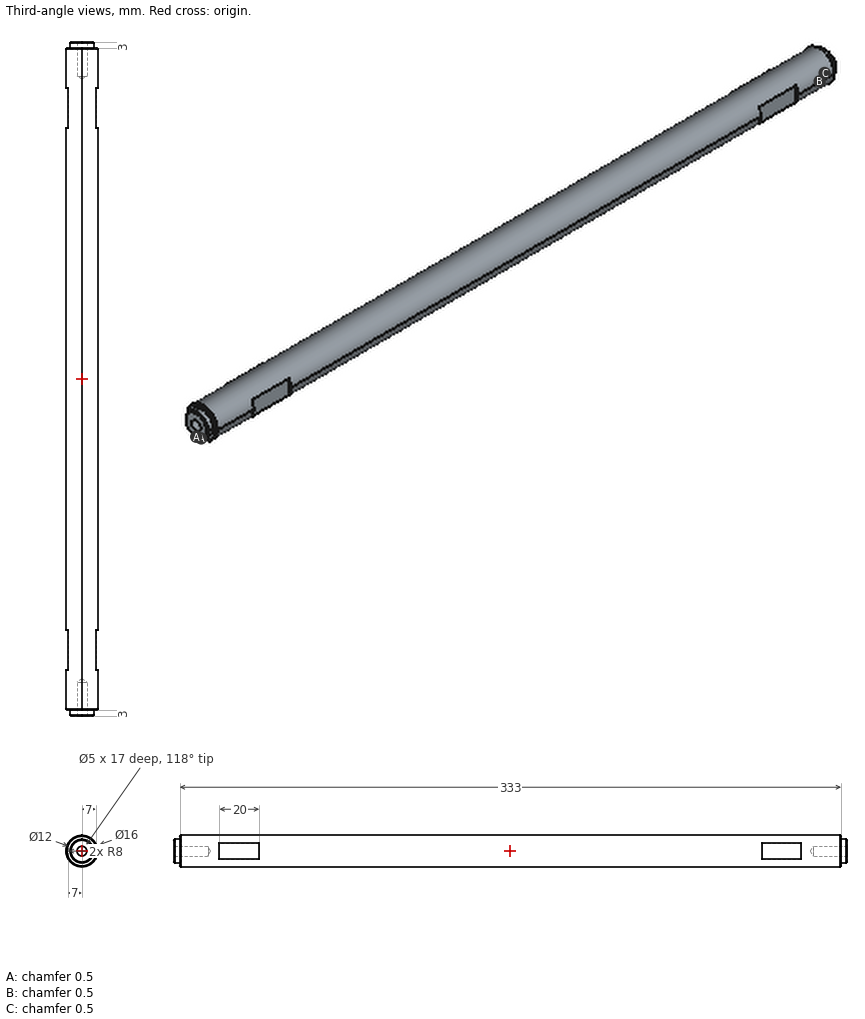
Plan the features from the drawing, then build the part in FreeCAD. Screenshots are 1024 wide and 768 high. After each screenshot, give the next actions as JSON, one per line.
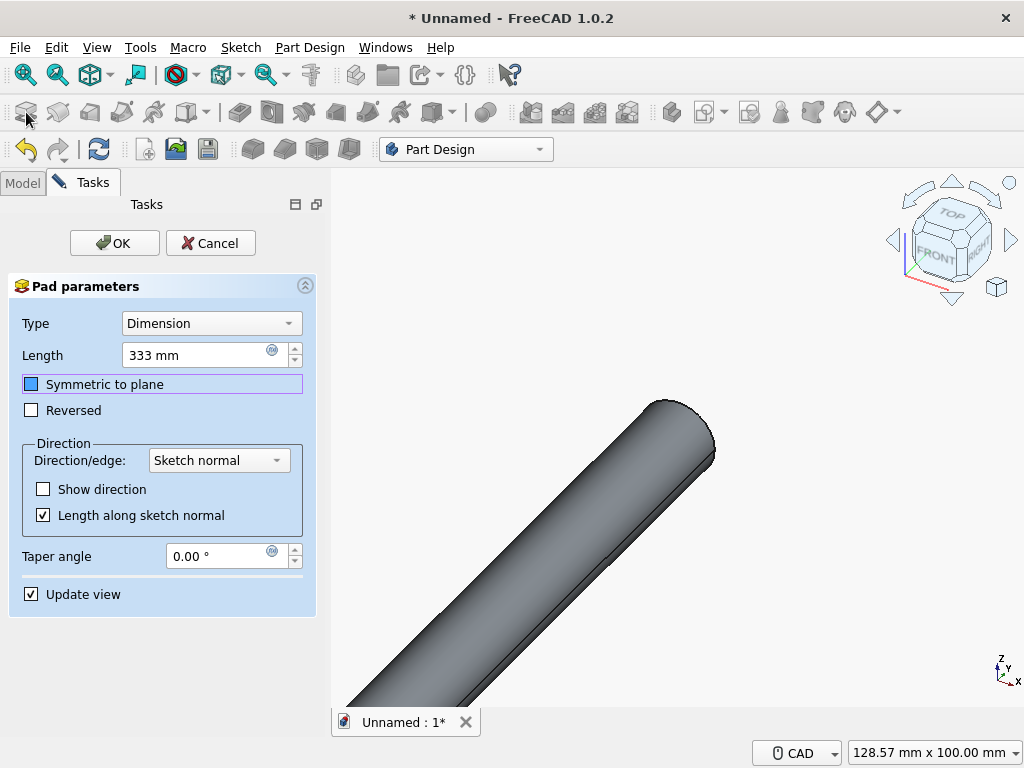
{"action": "left_click", "coordinate": [30, 384]}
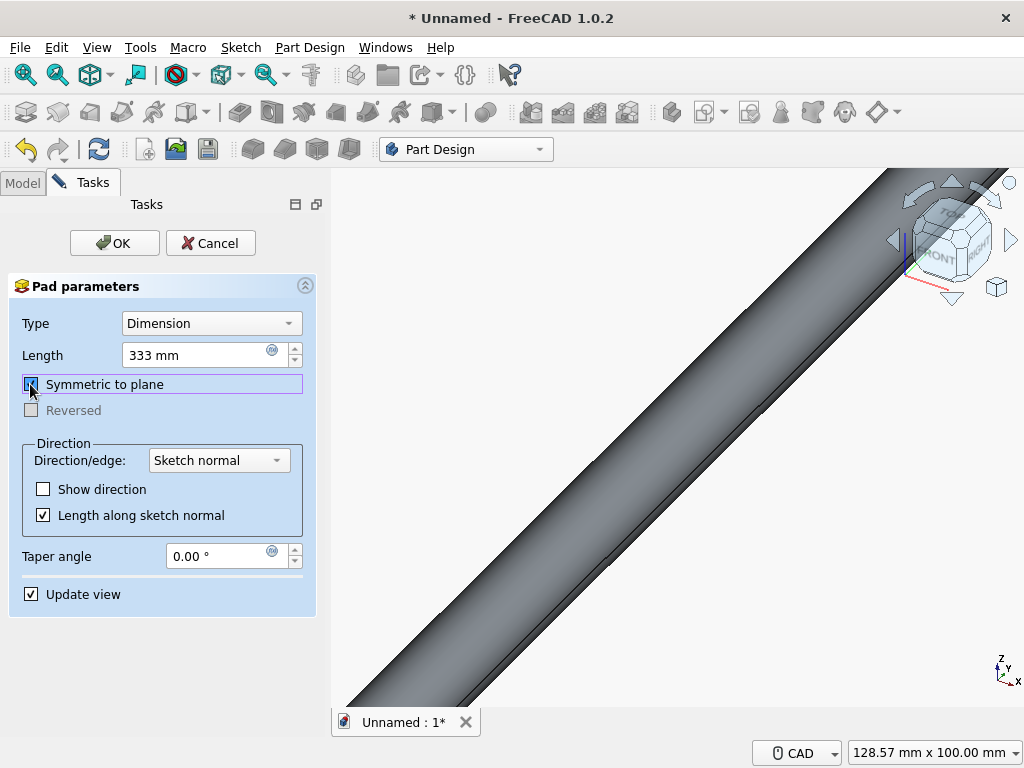
{"action": "left_click", "coordinate": [115, 243]}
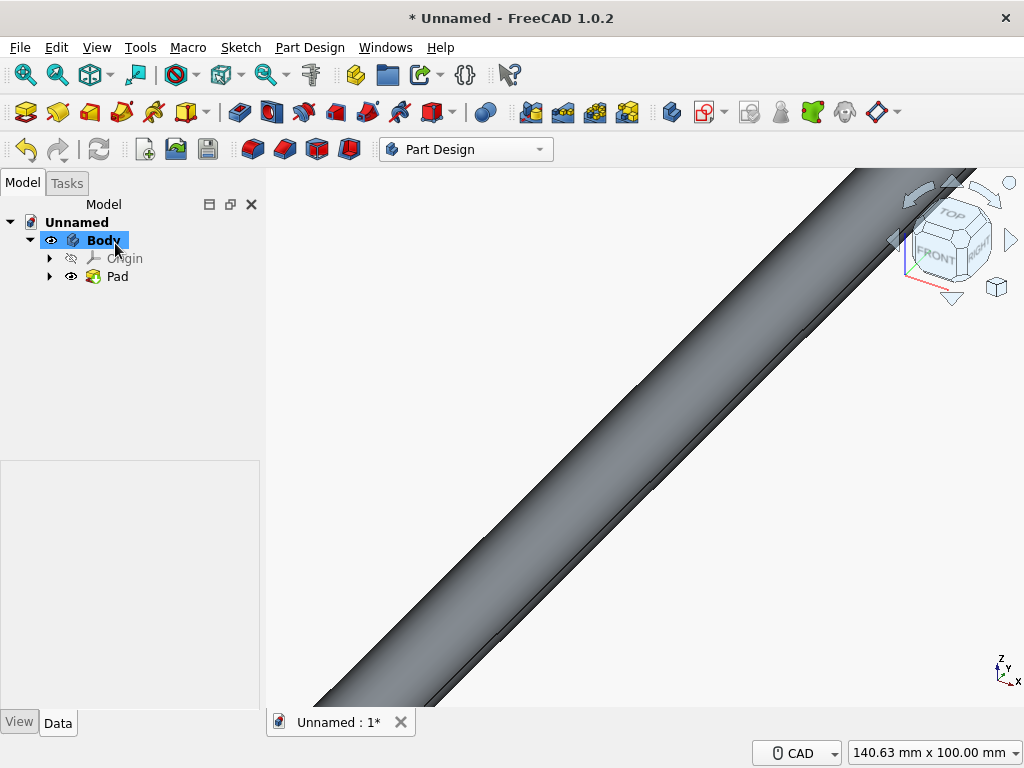
{"action": "left_click", "coordinate": [26, 76]}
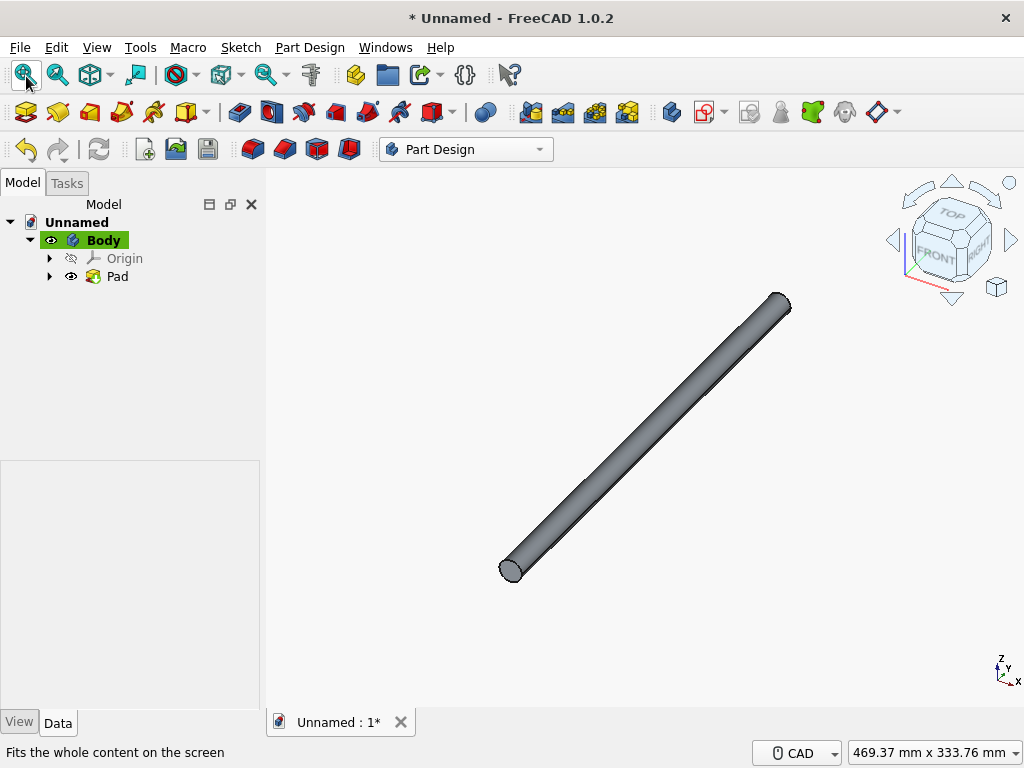
{"action": "left_click", "coordinate": [511, 573]}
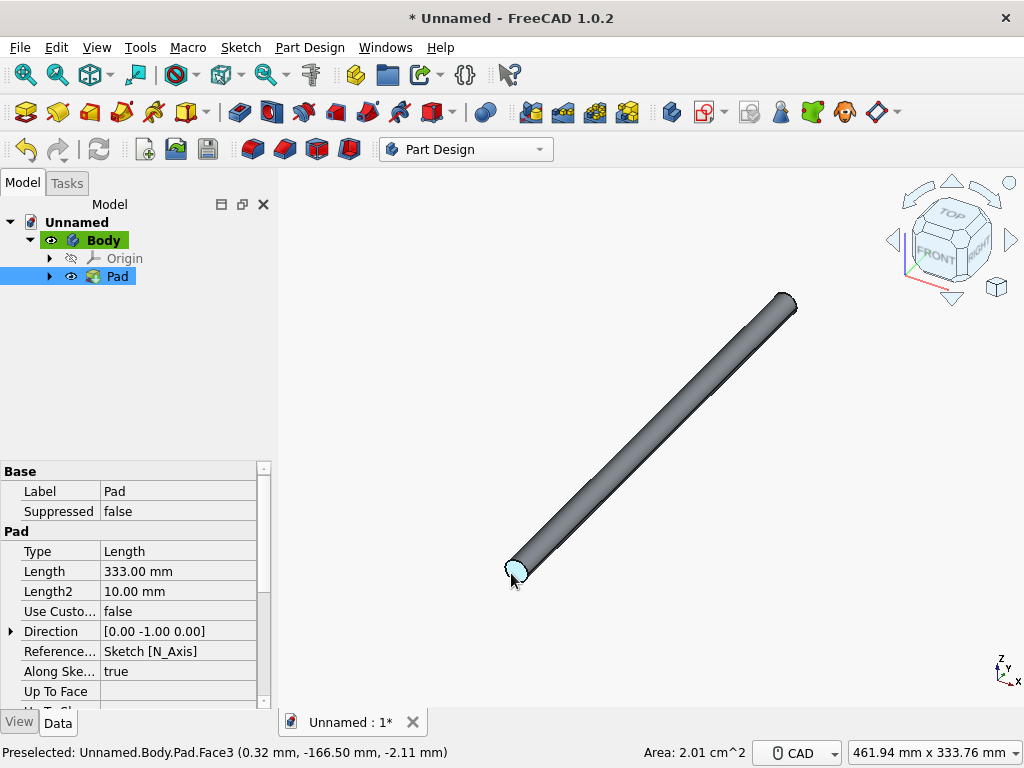
{"action": "left_click", "coordinate": [704, 112]}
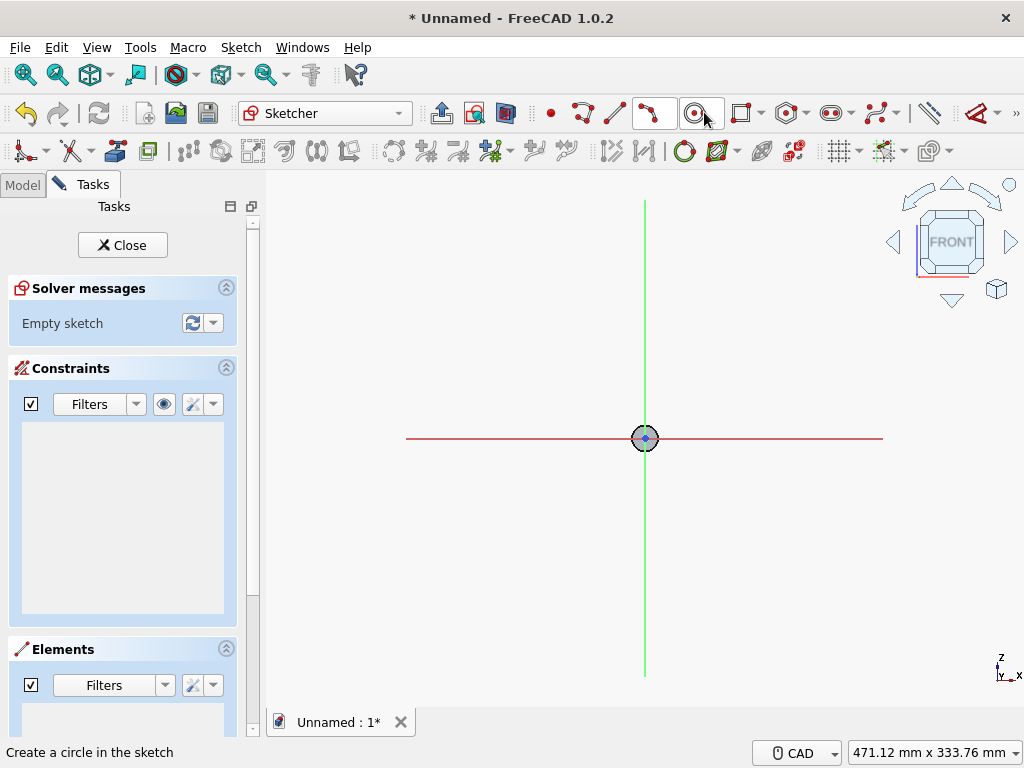
{"action": "scroll", "coordinate": [649, 438], "scroll_direction": "up", "scroll_amount": 14}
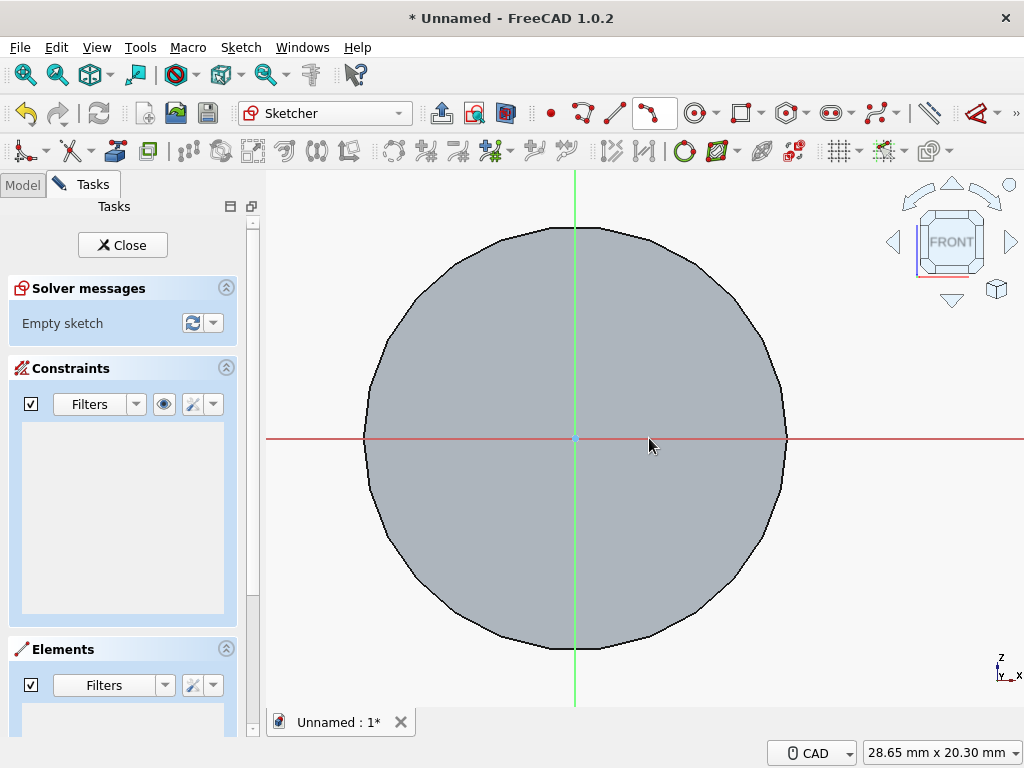
{"action": "key", "text": "g c"}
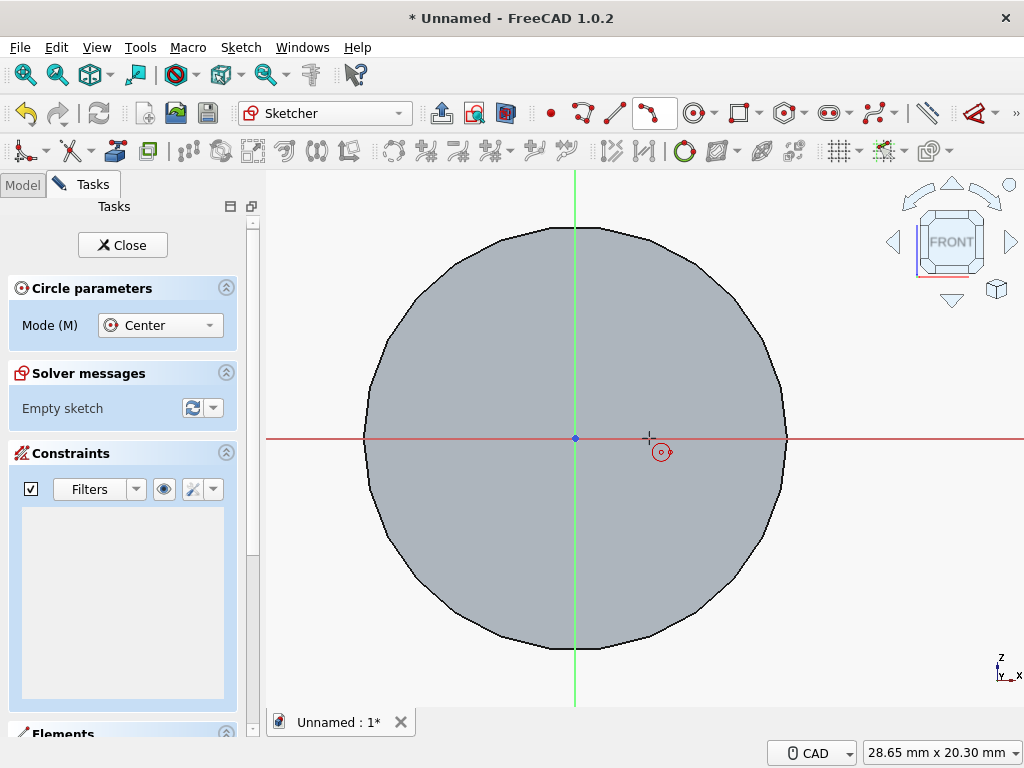
{"action": "left_click", "coordinate": [575, 438]}
{"action": "left_click", "coordinate": [688, 326]}
{"action": "key", "text": "Escape"}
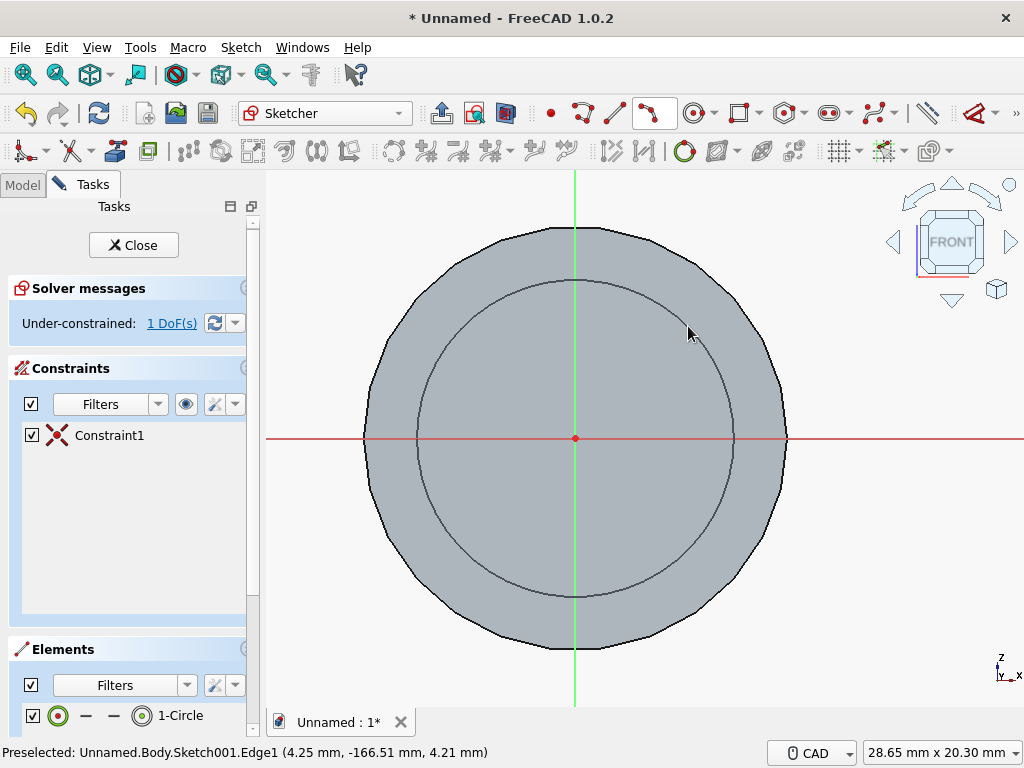
{"action": "key", "text": "d"}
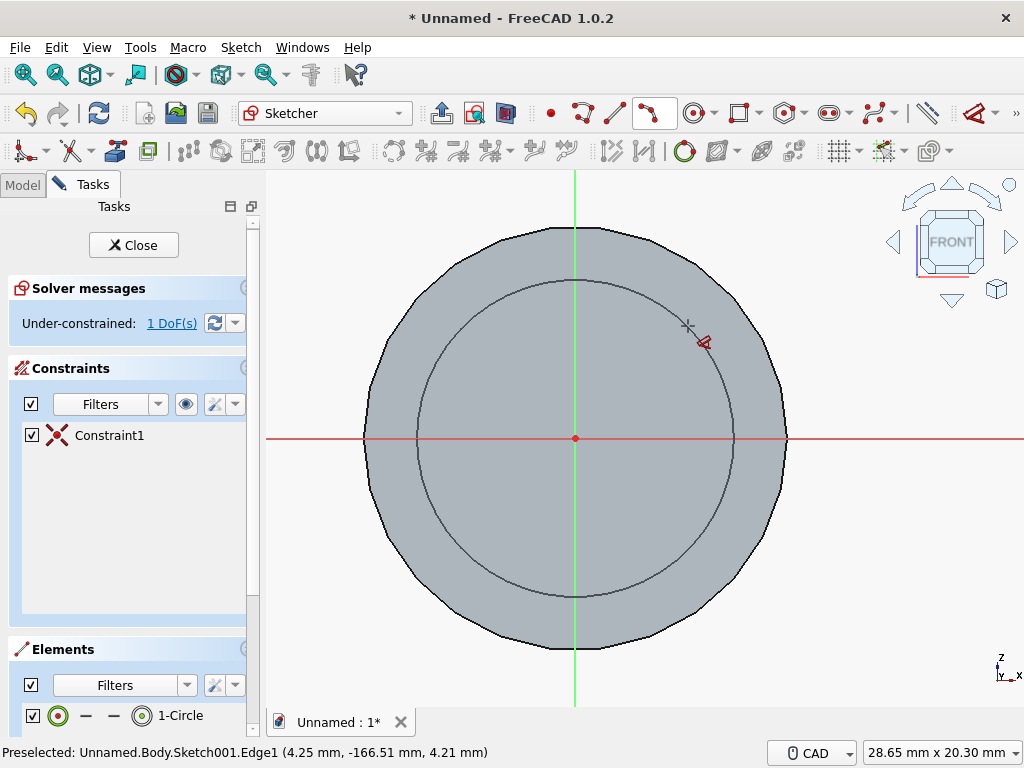
{"action": "left_click", "coordinate": [687, 326]}
{"action": "left_click", "coordinate": [710, 303]}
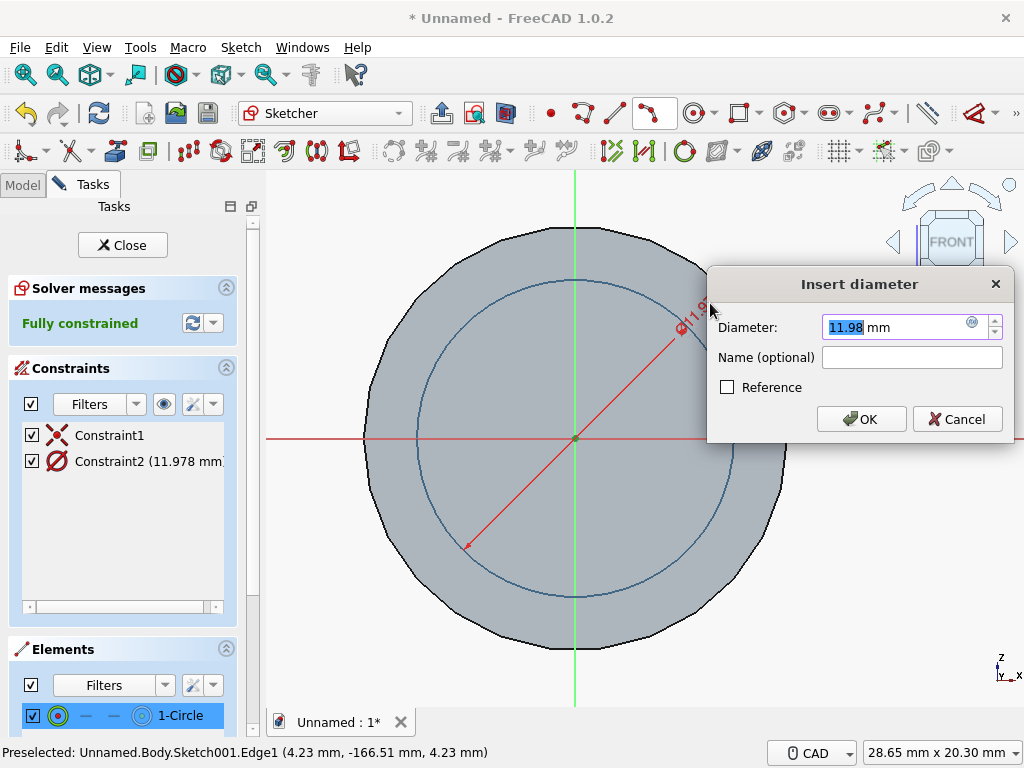
{"action": "type", "text": "12"}
{"action": "key", "text": "Return"}
{"action": "key", "text": "Escape"}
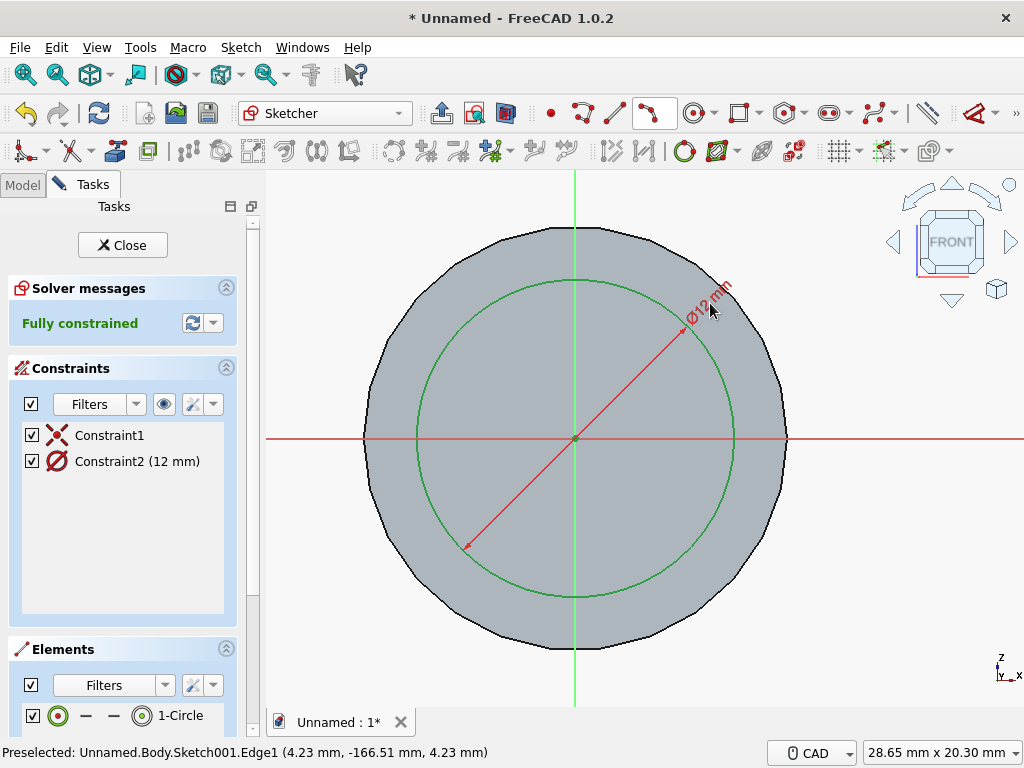
{"action": "left_click", "coordinate": [123, 245]}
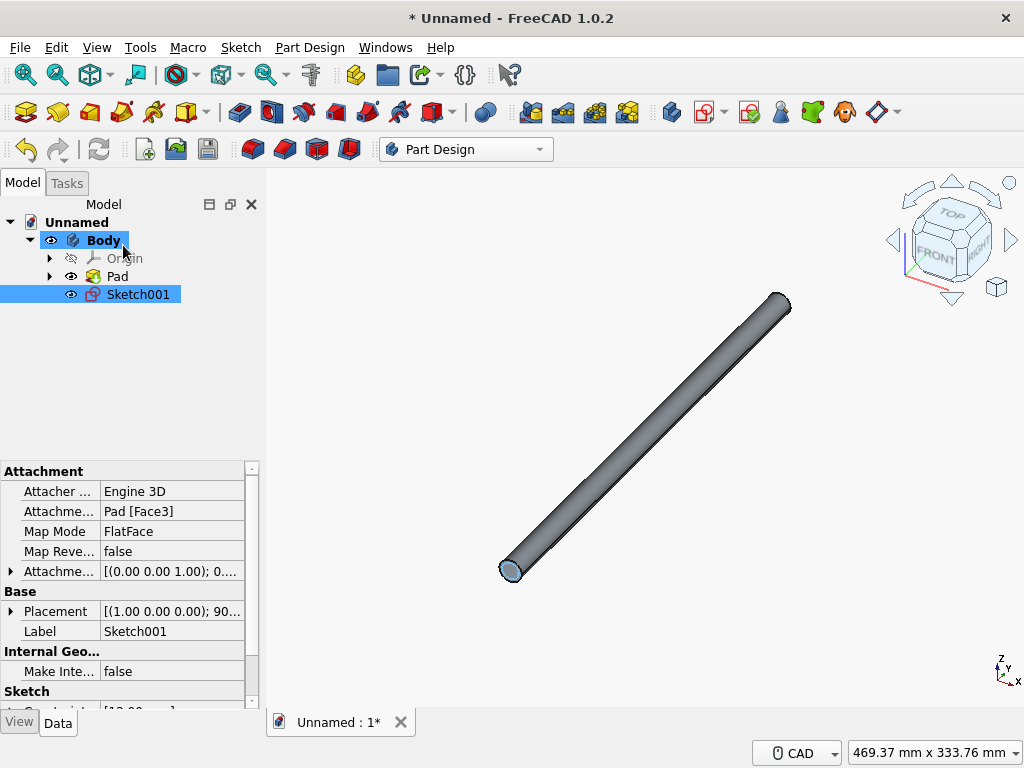
{"action": "left_click", "coordinate": [26, 112]}